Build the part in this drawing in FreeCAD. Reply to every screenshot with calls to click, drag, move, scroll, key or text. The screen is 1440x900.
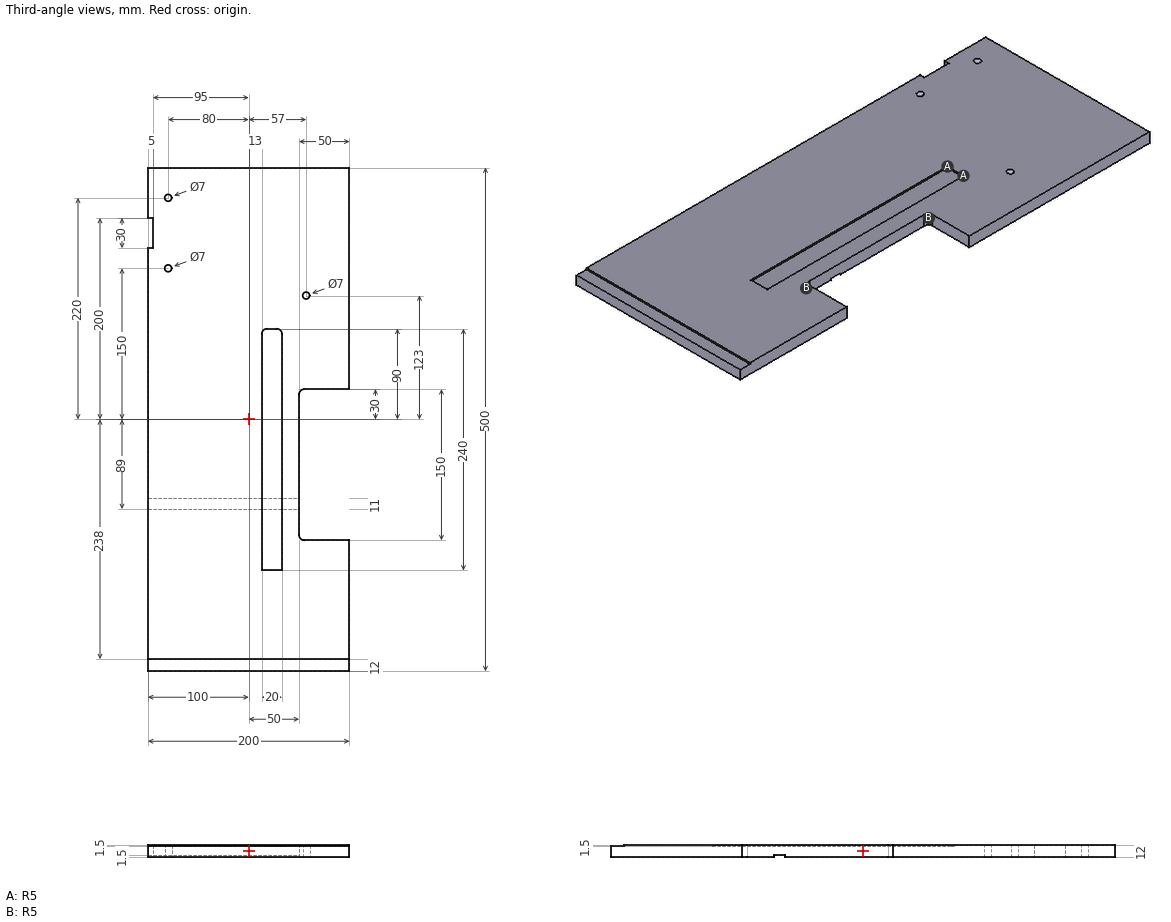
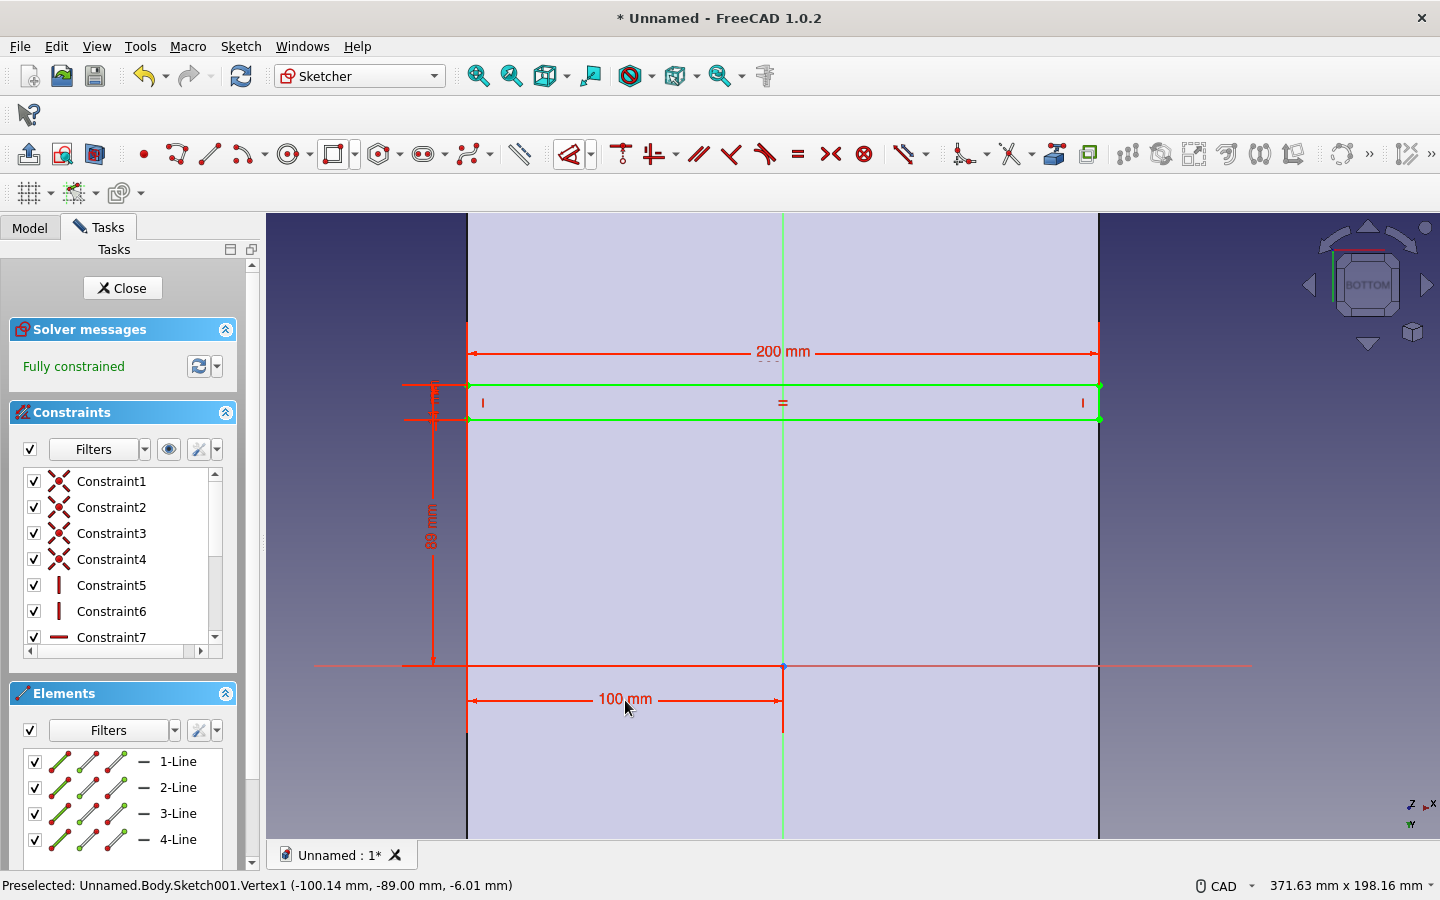
click(123, 288)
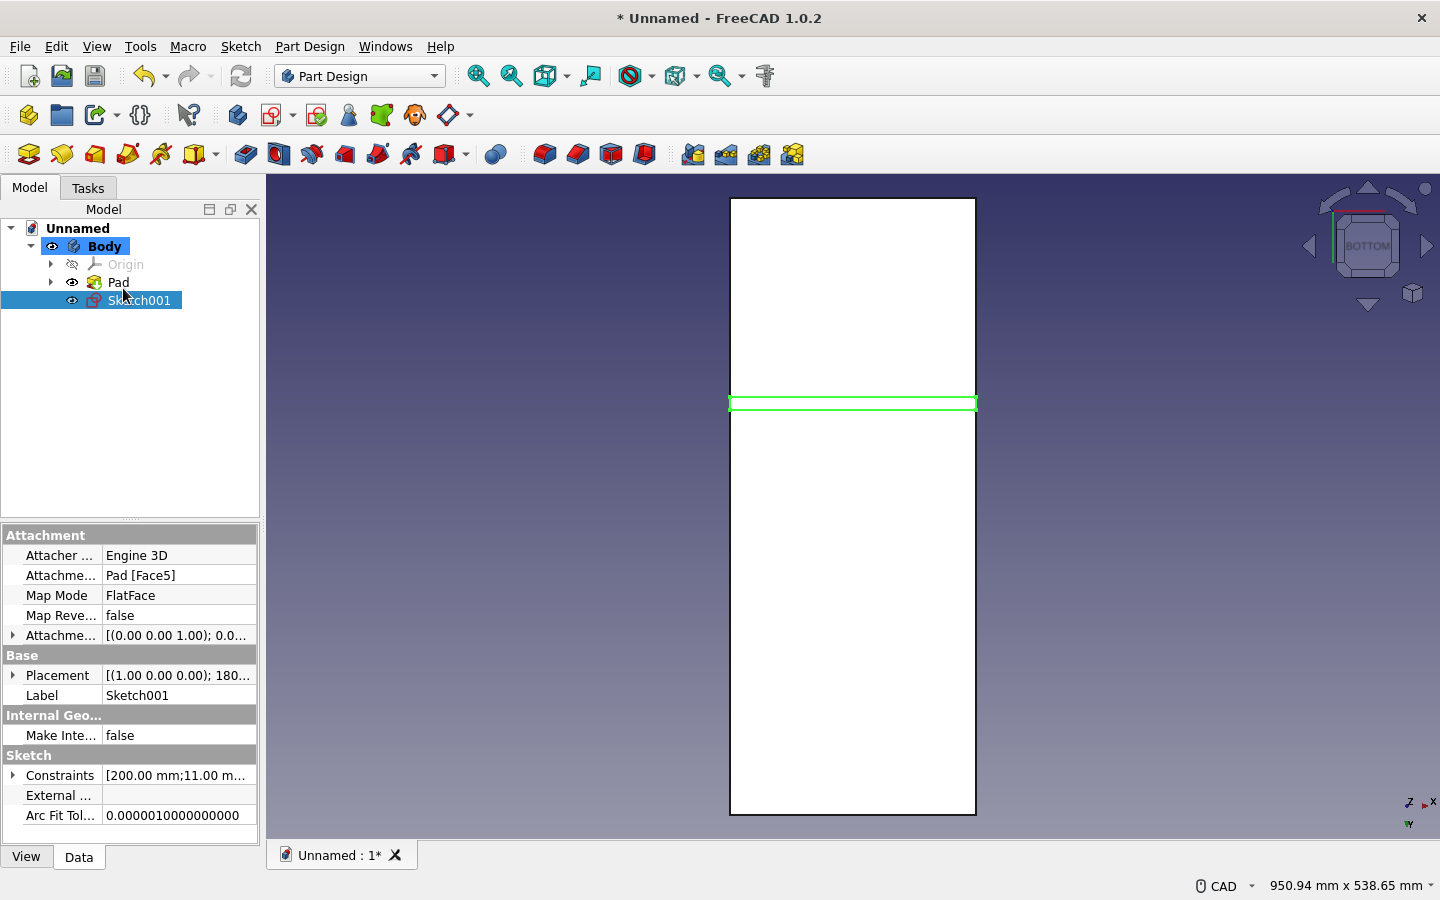
click(246, 154)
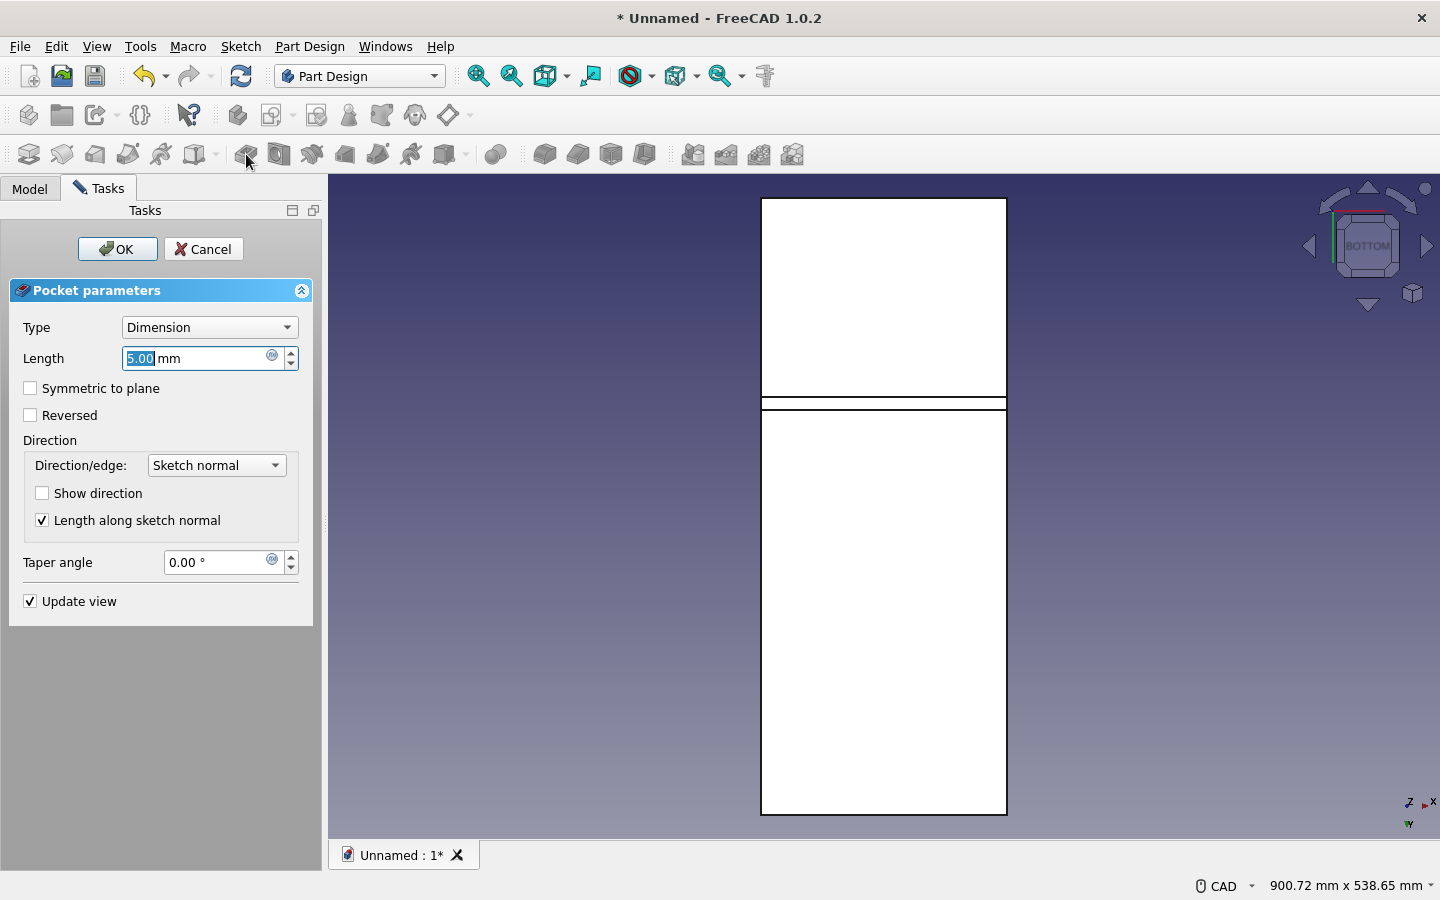
text(1.5)
key(Tab)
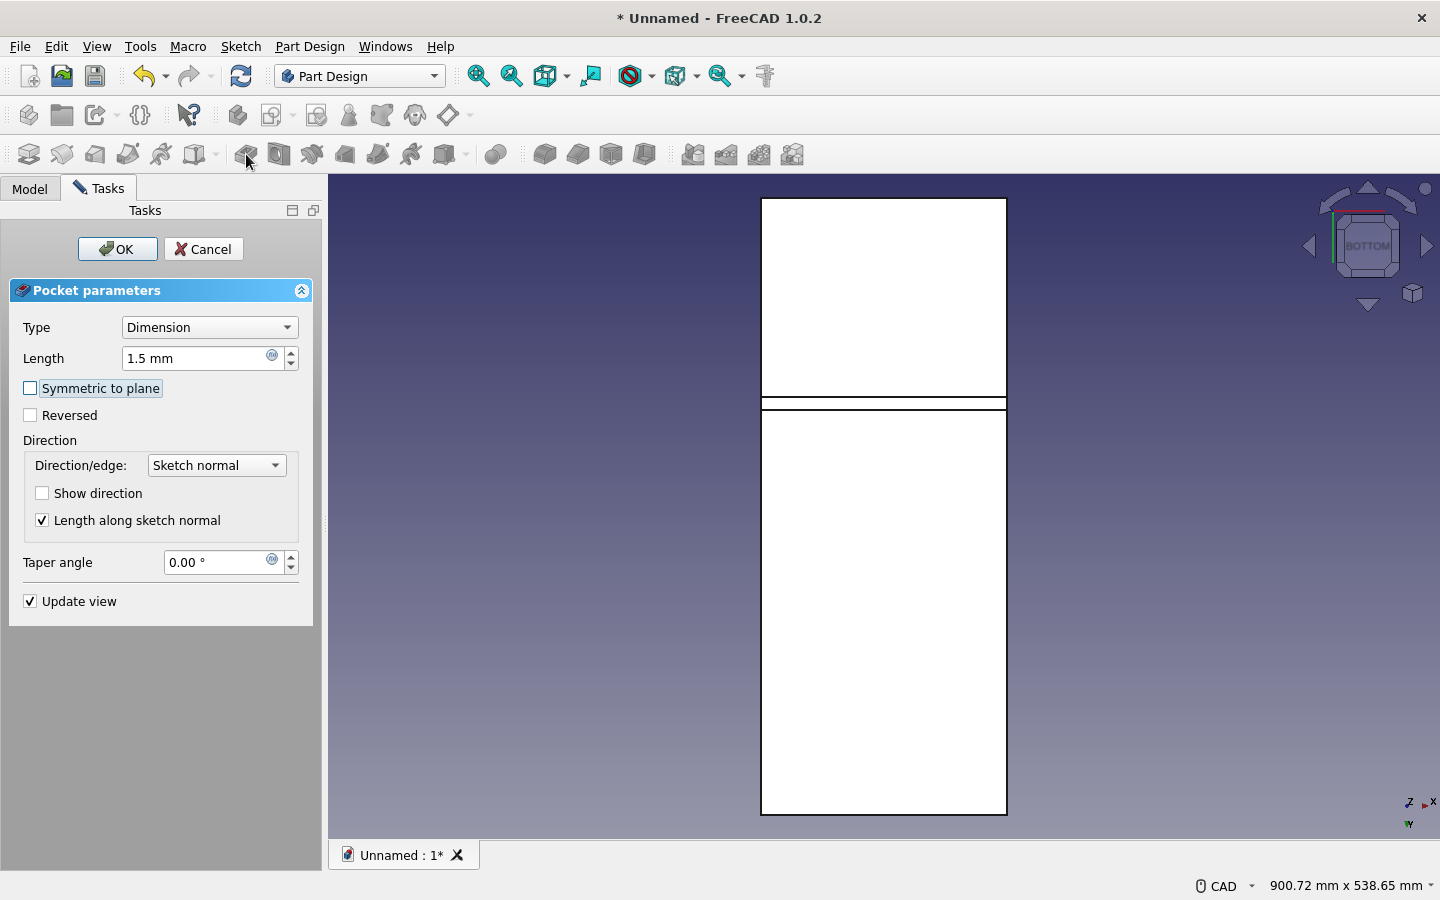
click(118, 249)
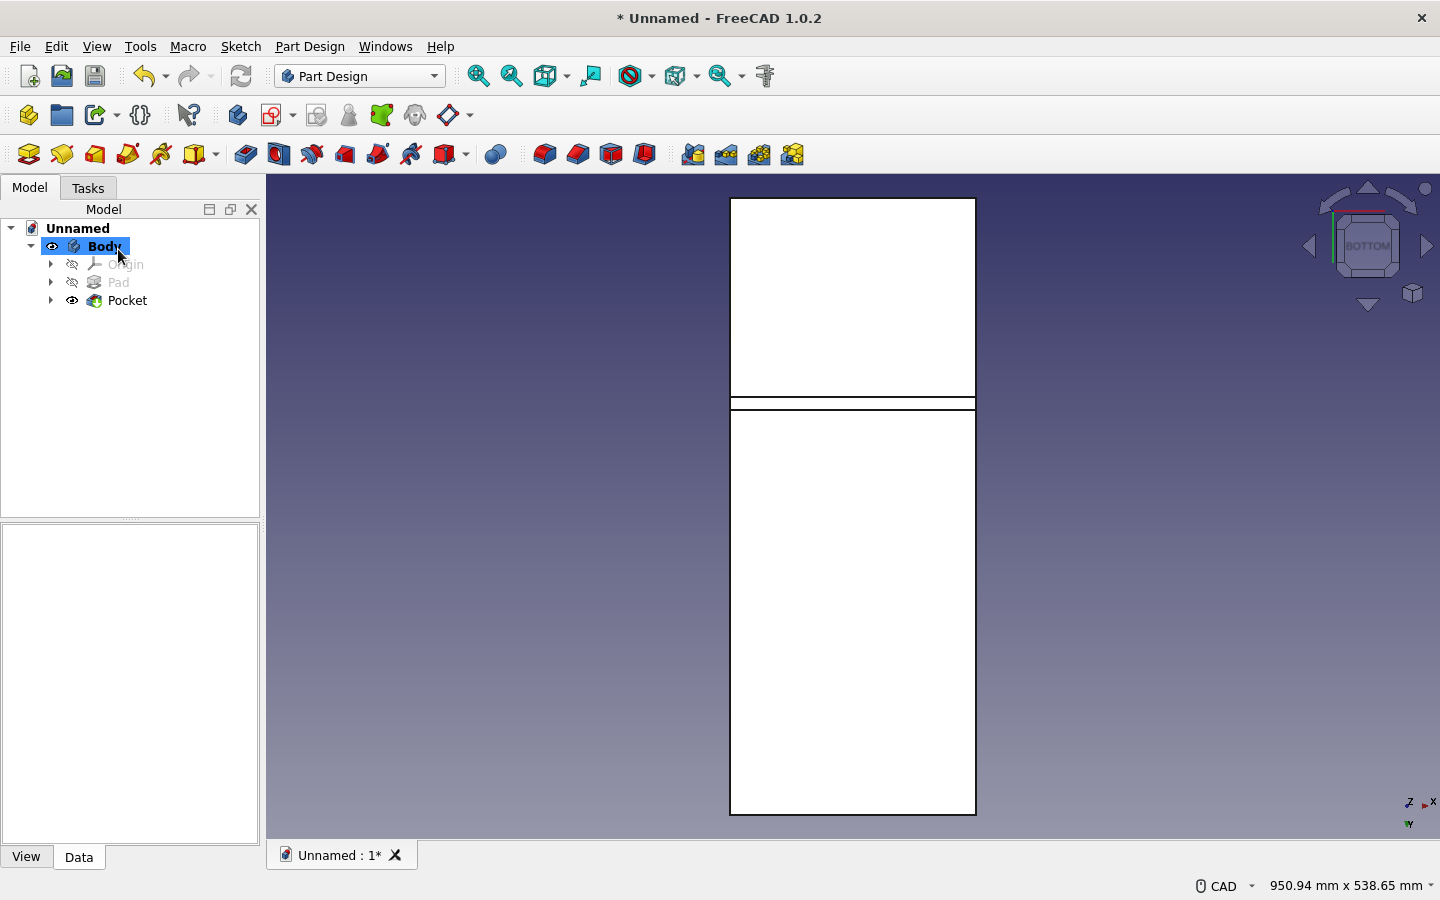
key(0)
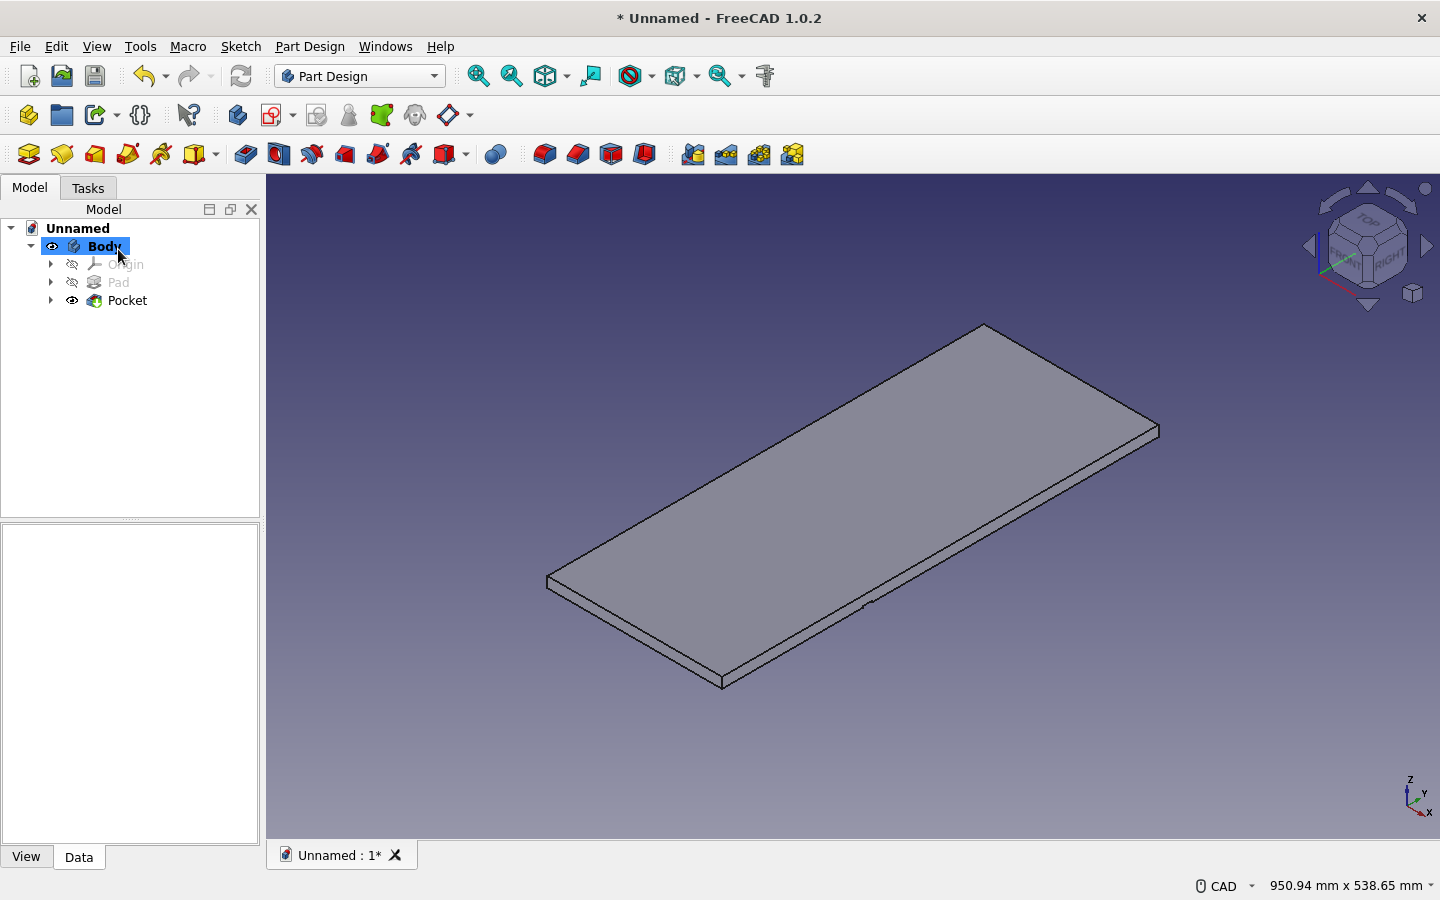
click(978, 427)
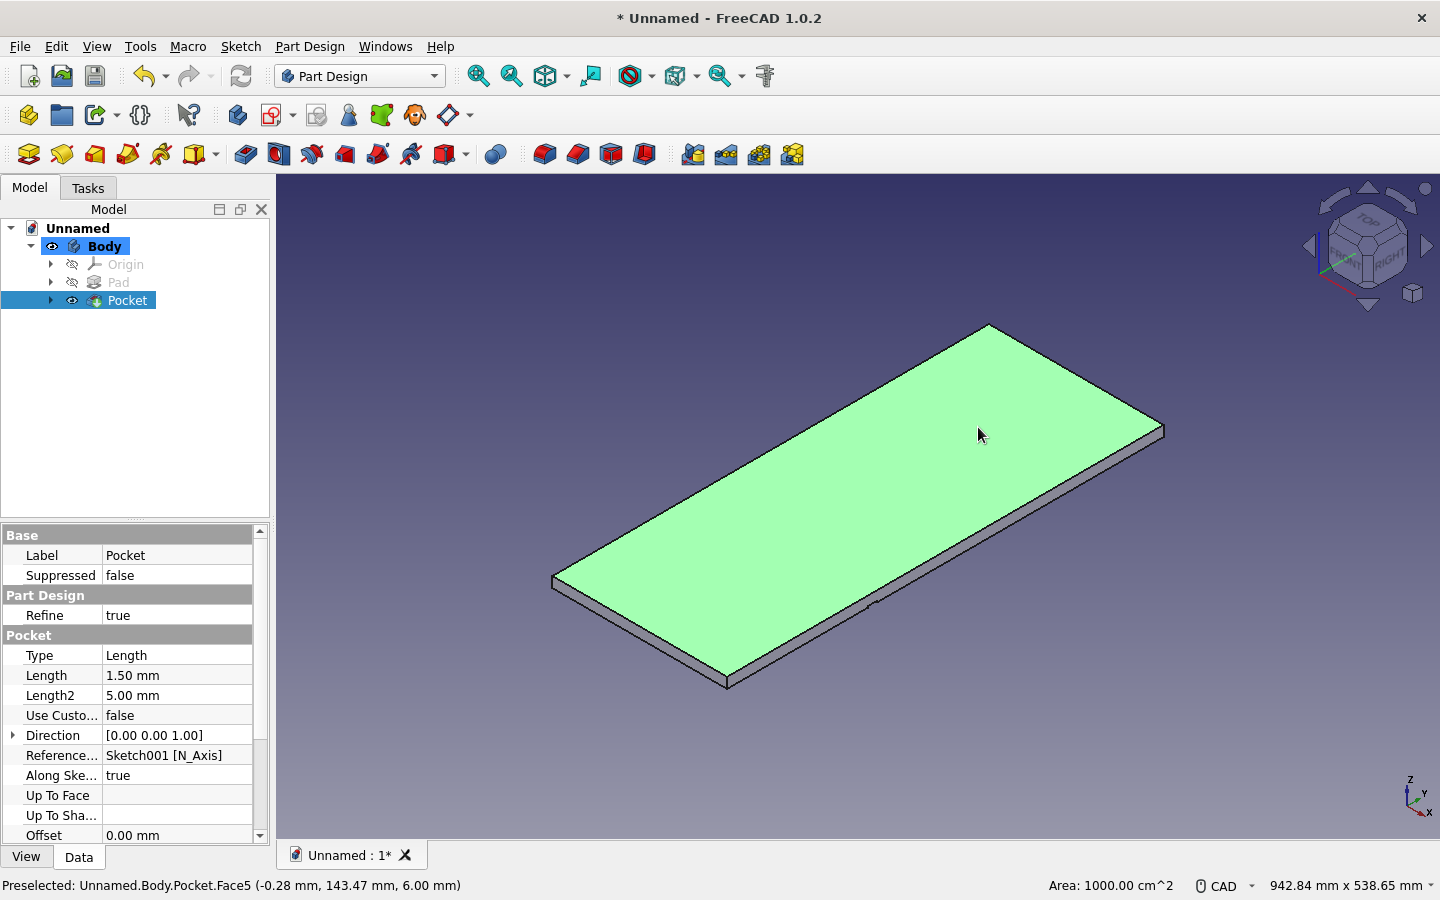
click(270, 116)